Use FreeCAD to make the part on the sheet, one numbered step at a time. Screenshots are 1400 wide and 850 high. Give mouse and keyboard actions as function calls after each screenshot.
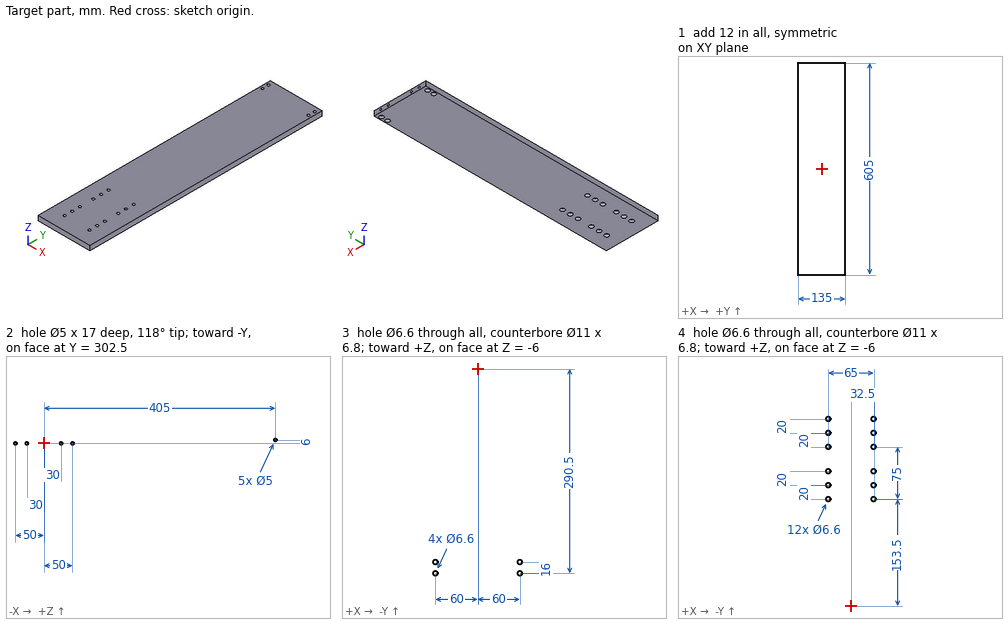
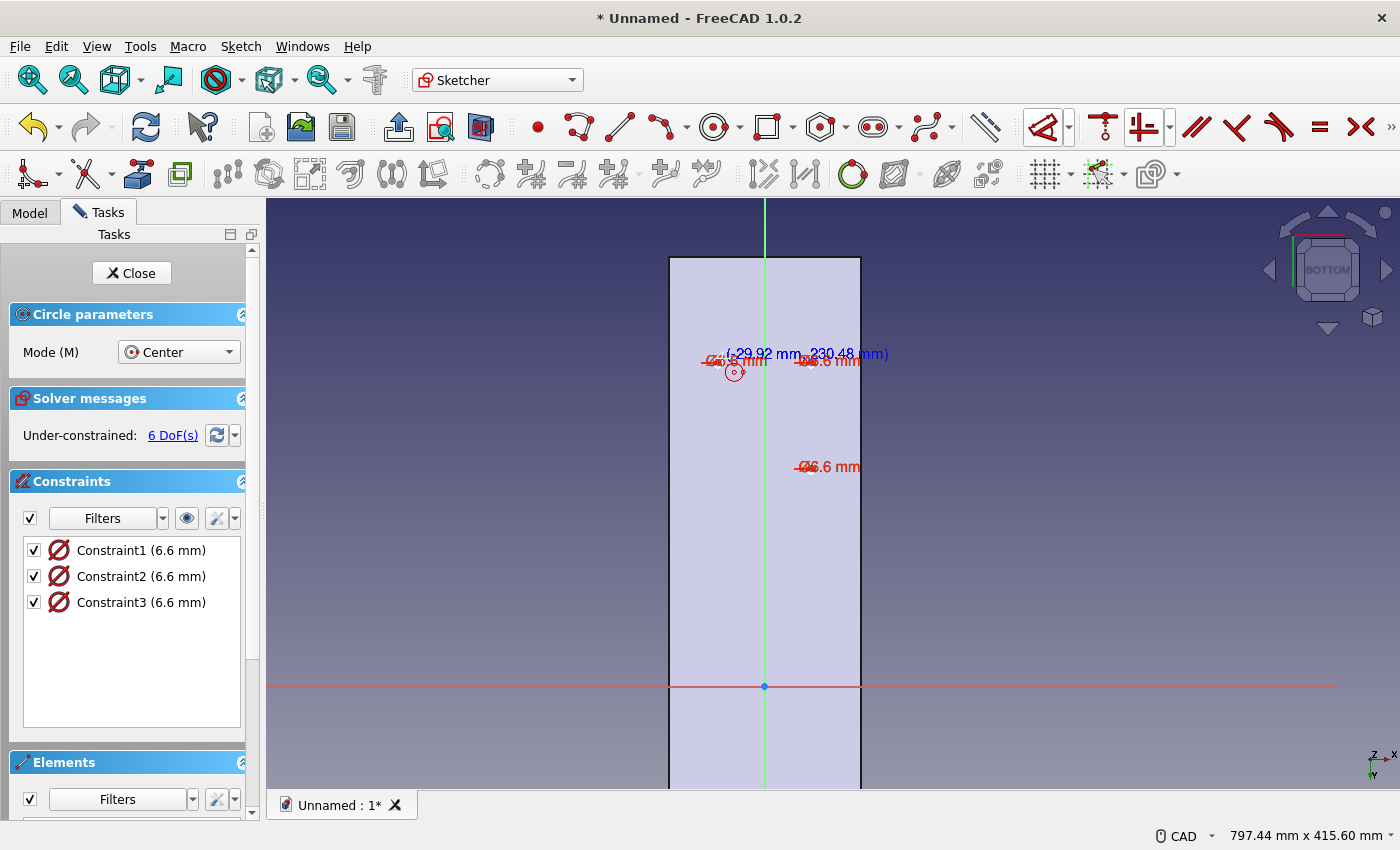
scroll(718, 468, up, 8)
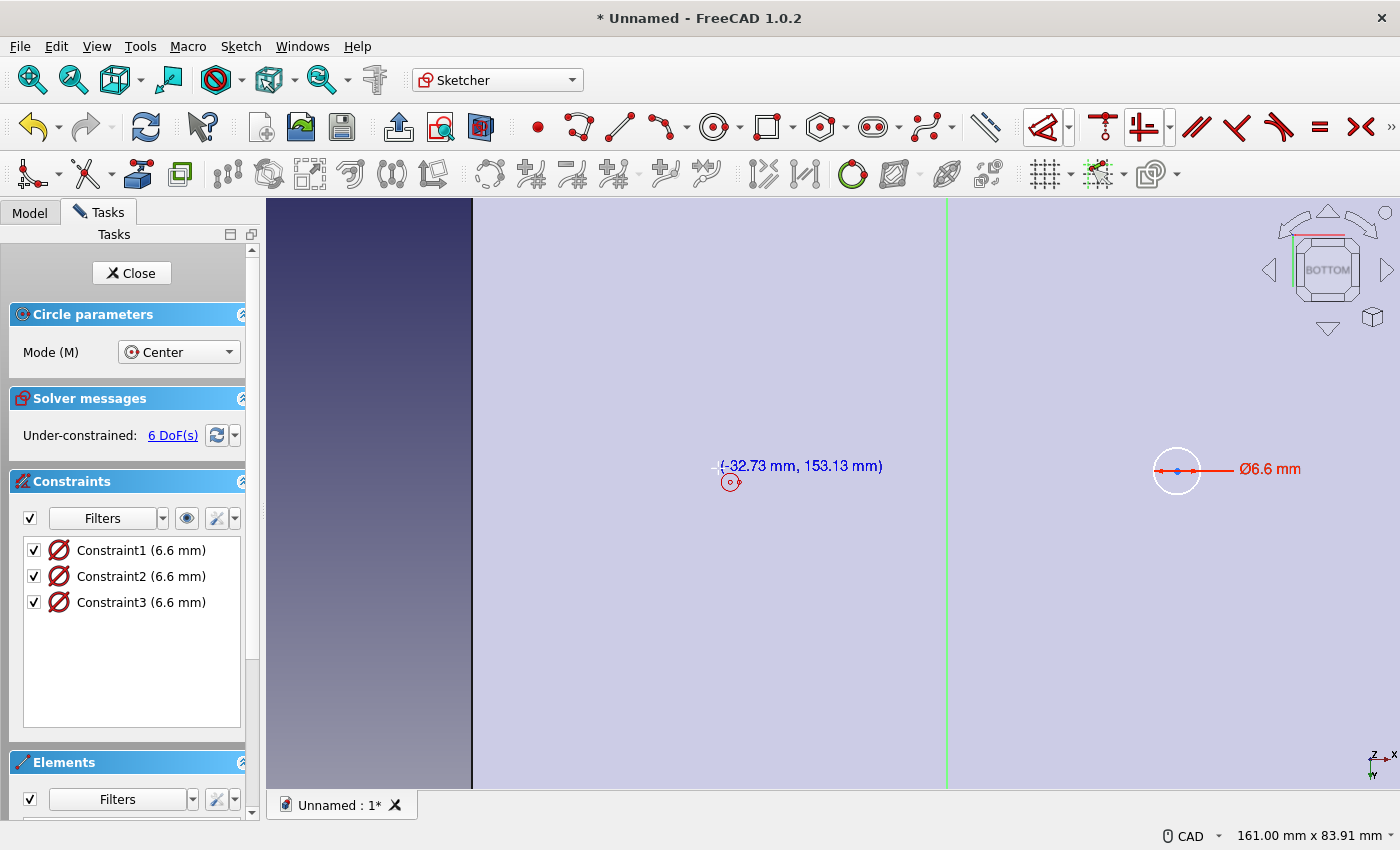
scroll(718, 468, down, 8)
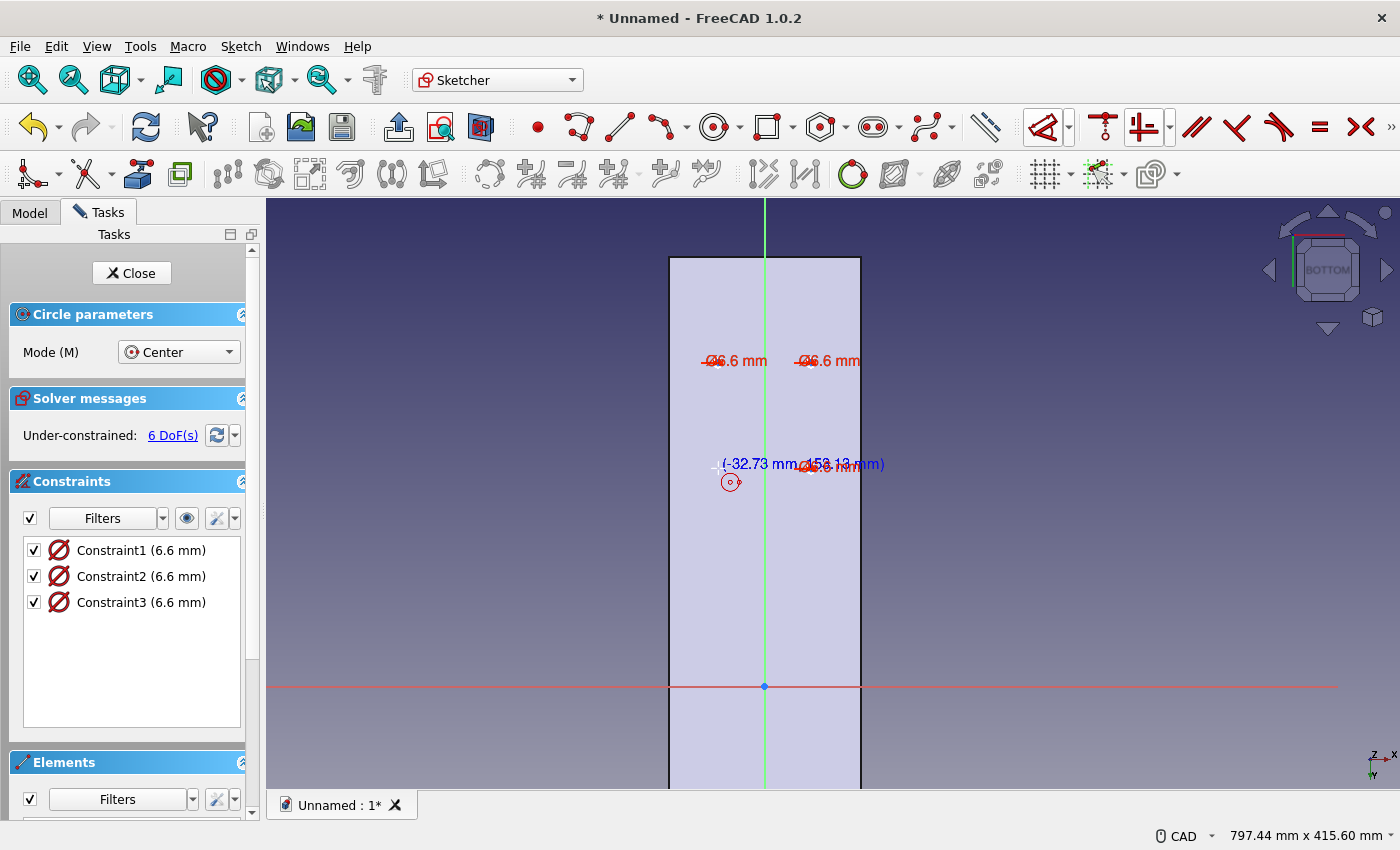
click(718, 468)
move(722, 465)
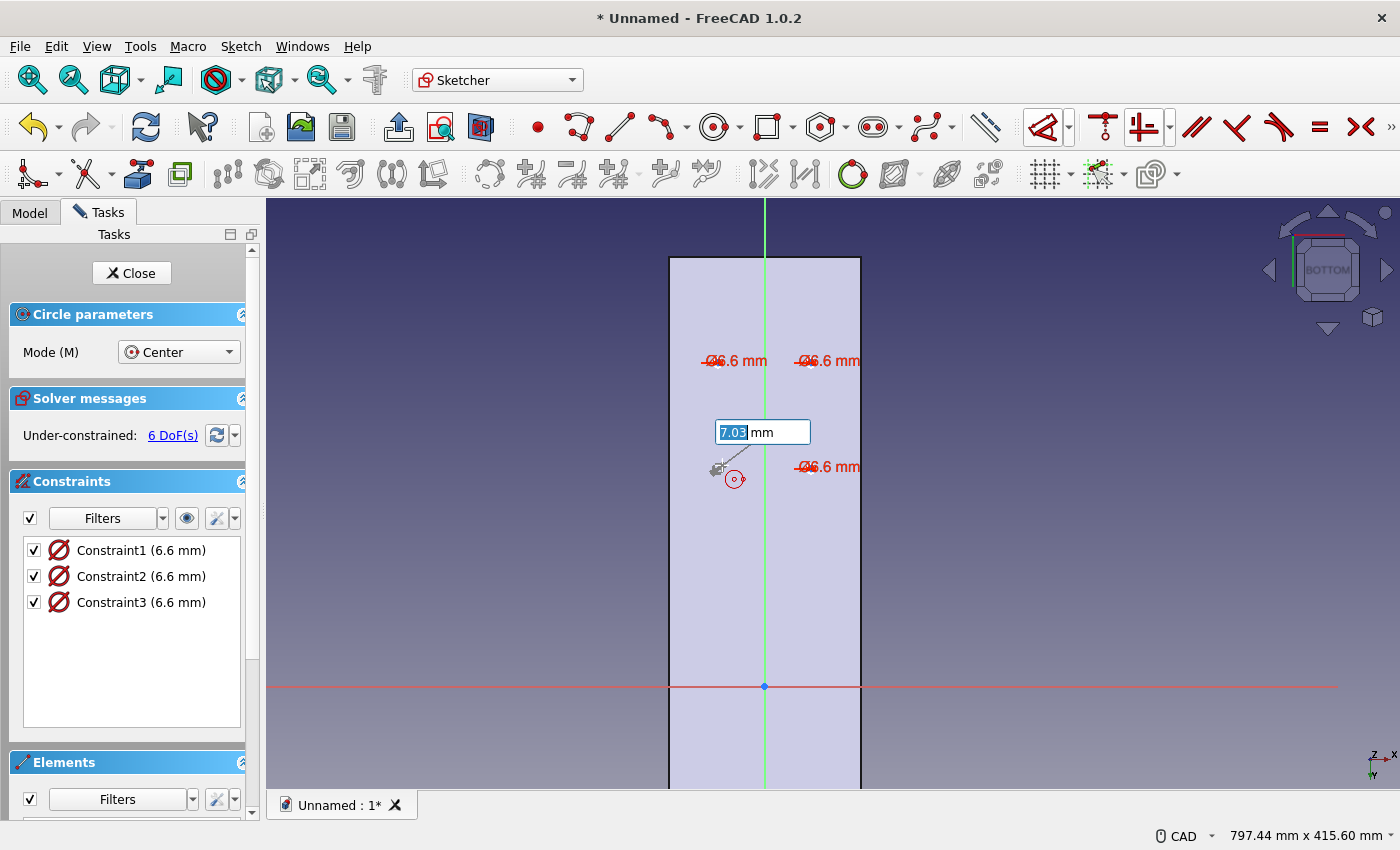
text(6.6)
key(Return)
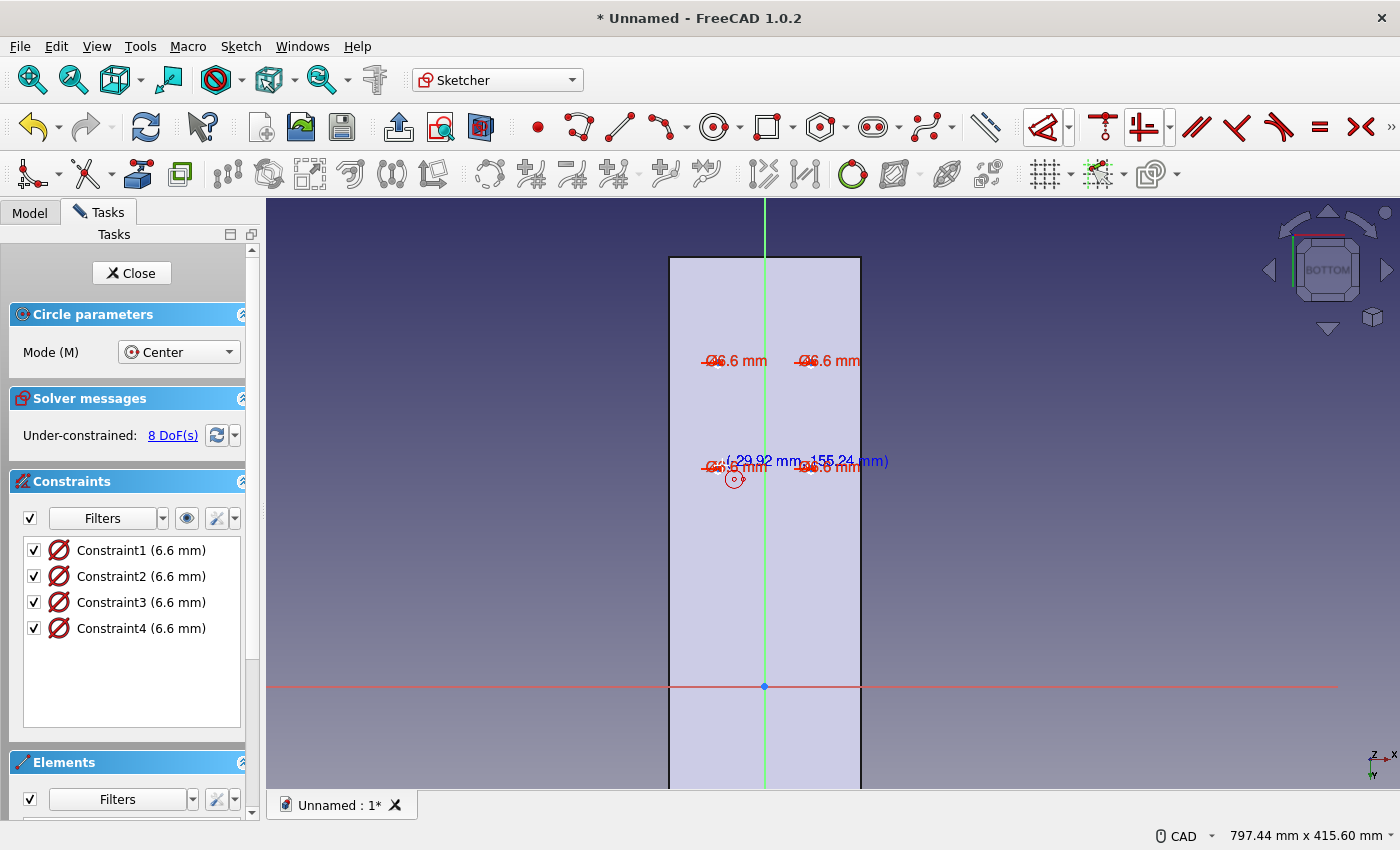
scroll(718, 440, up, 8)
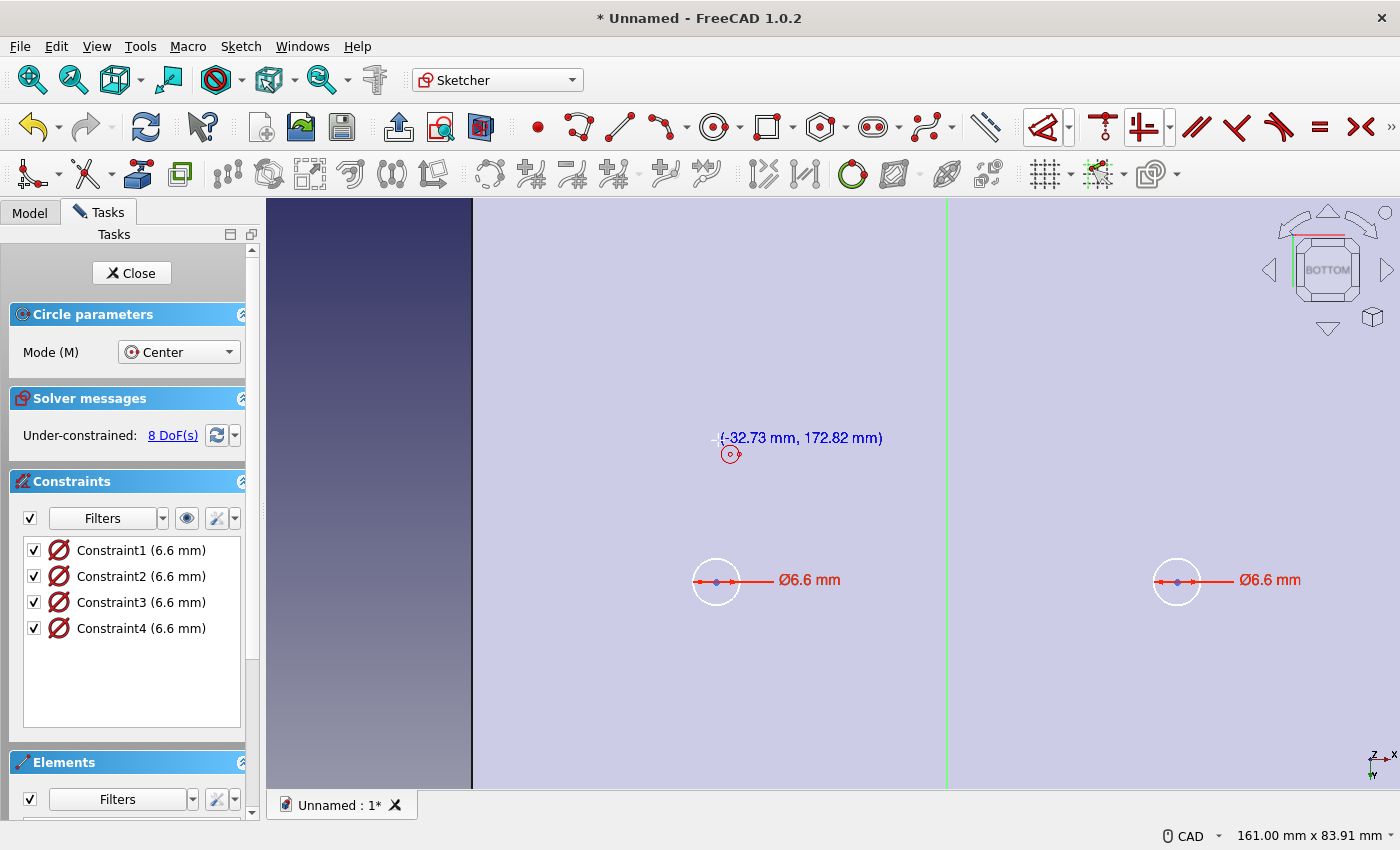
scroll(718, 440, down, 8)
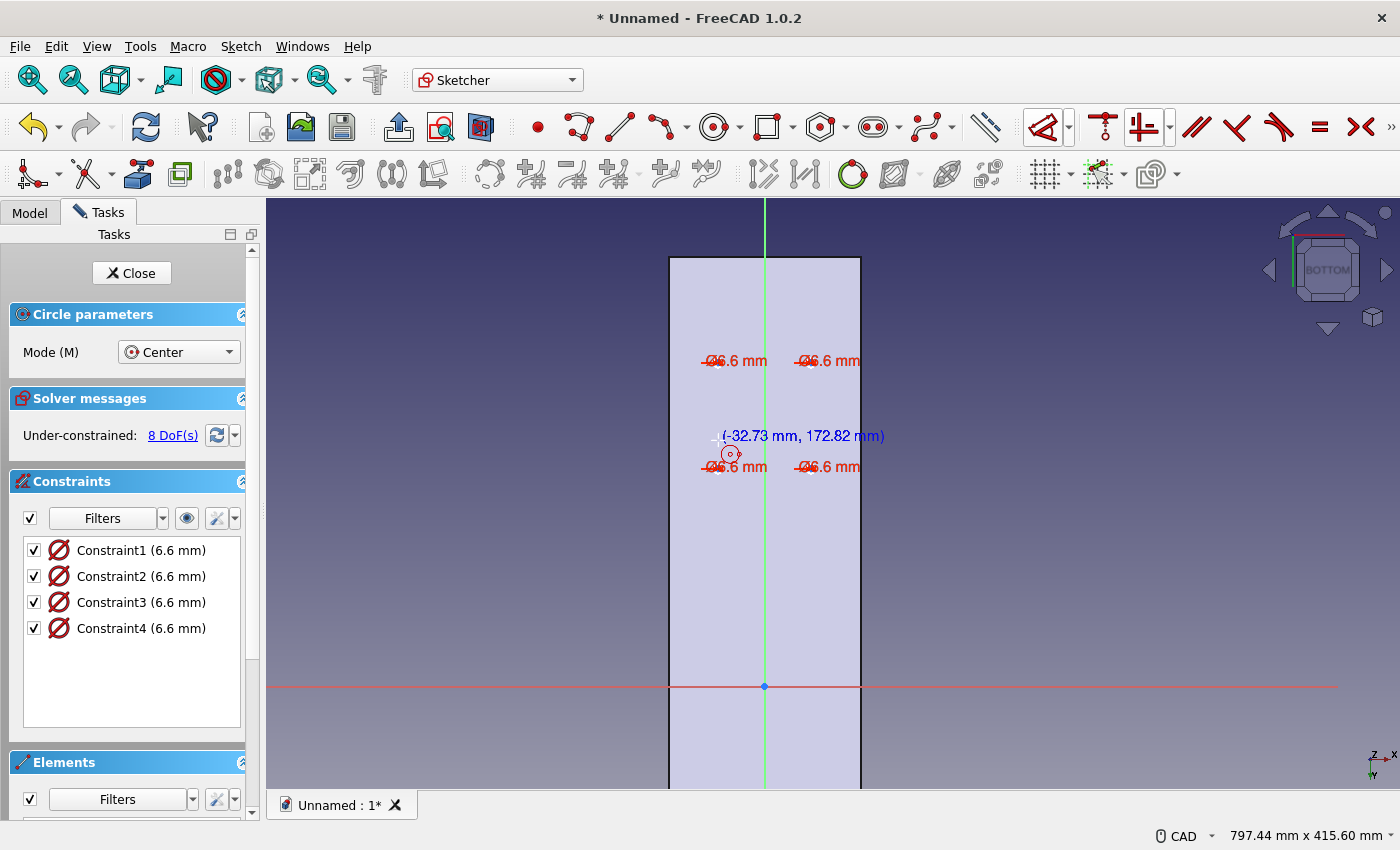
click(718, 440)
move(722, 437)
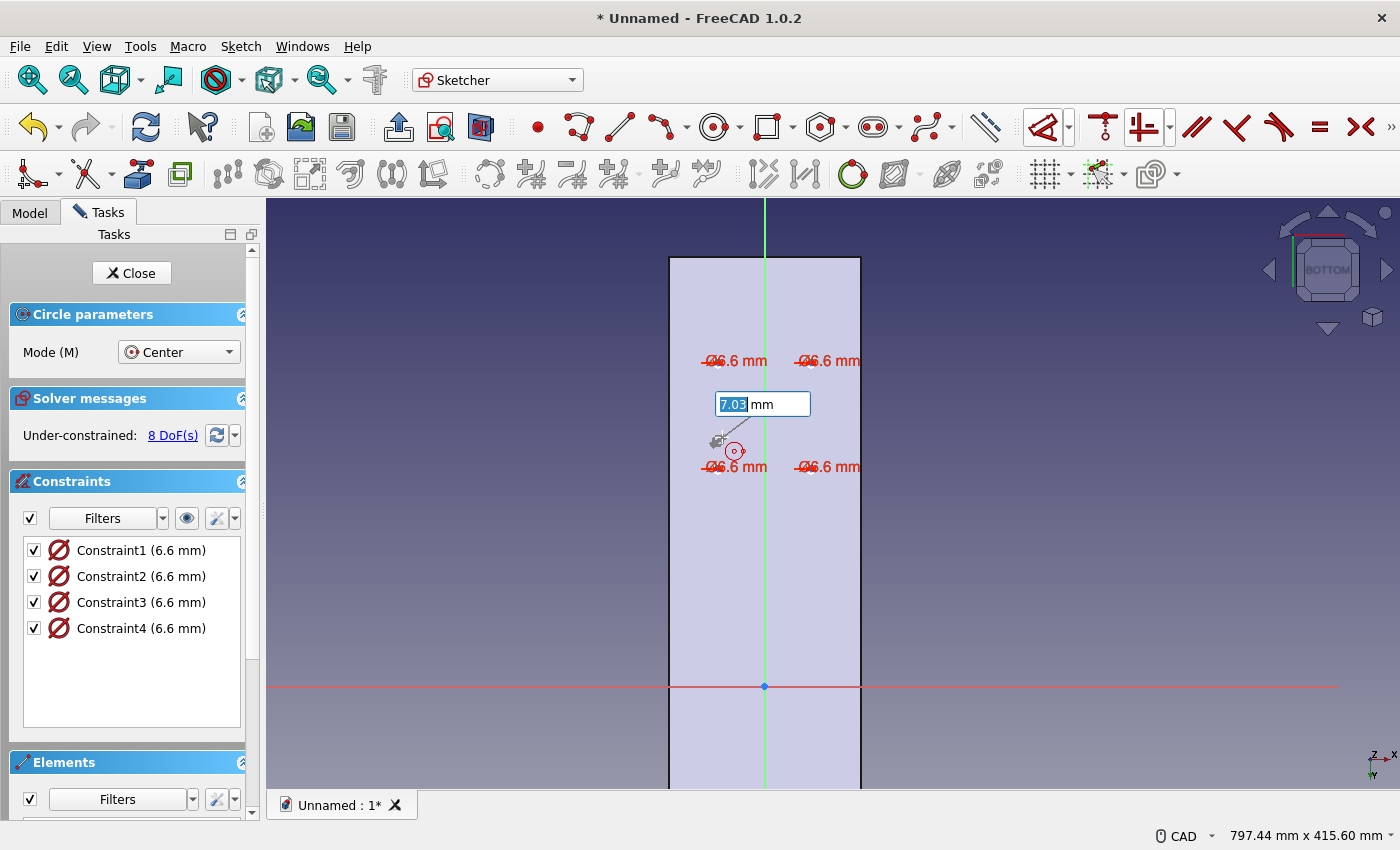
text(6.6)
key(Return)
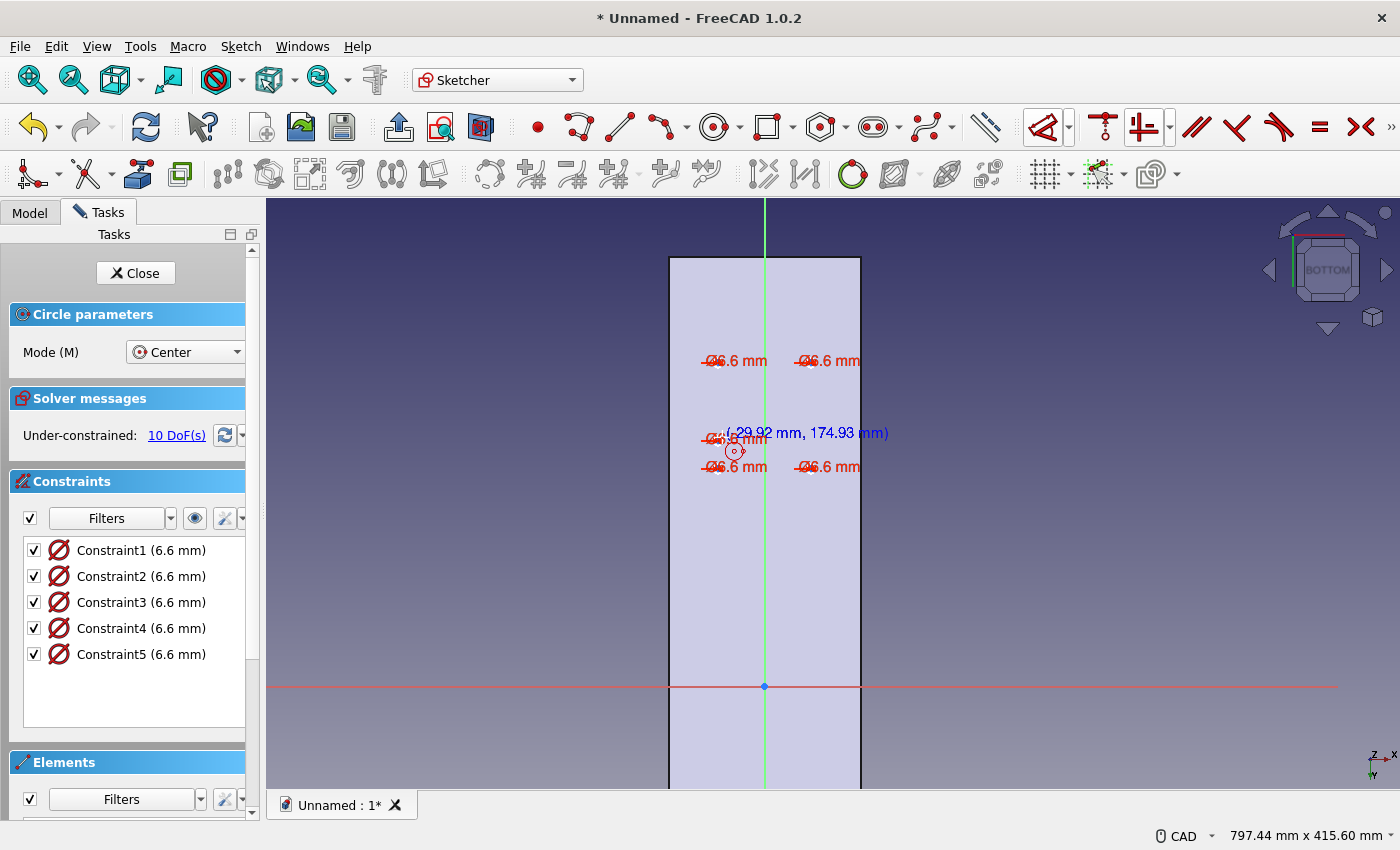
scroll(718, 333, up, 8)